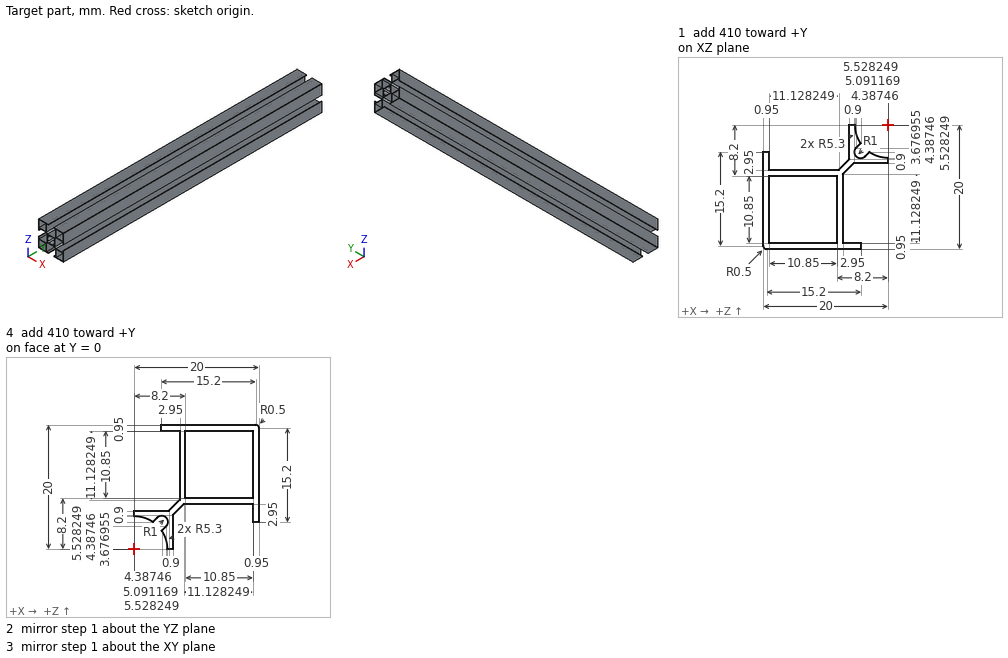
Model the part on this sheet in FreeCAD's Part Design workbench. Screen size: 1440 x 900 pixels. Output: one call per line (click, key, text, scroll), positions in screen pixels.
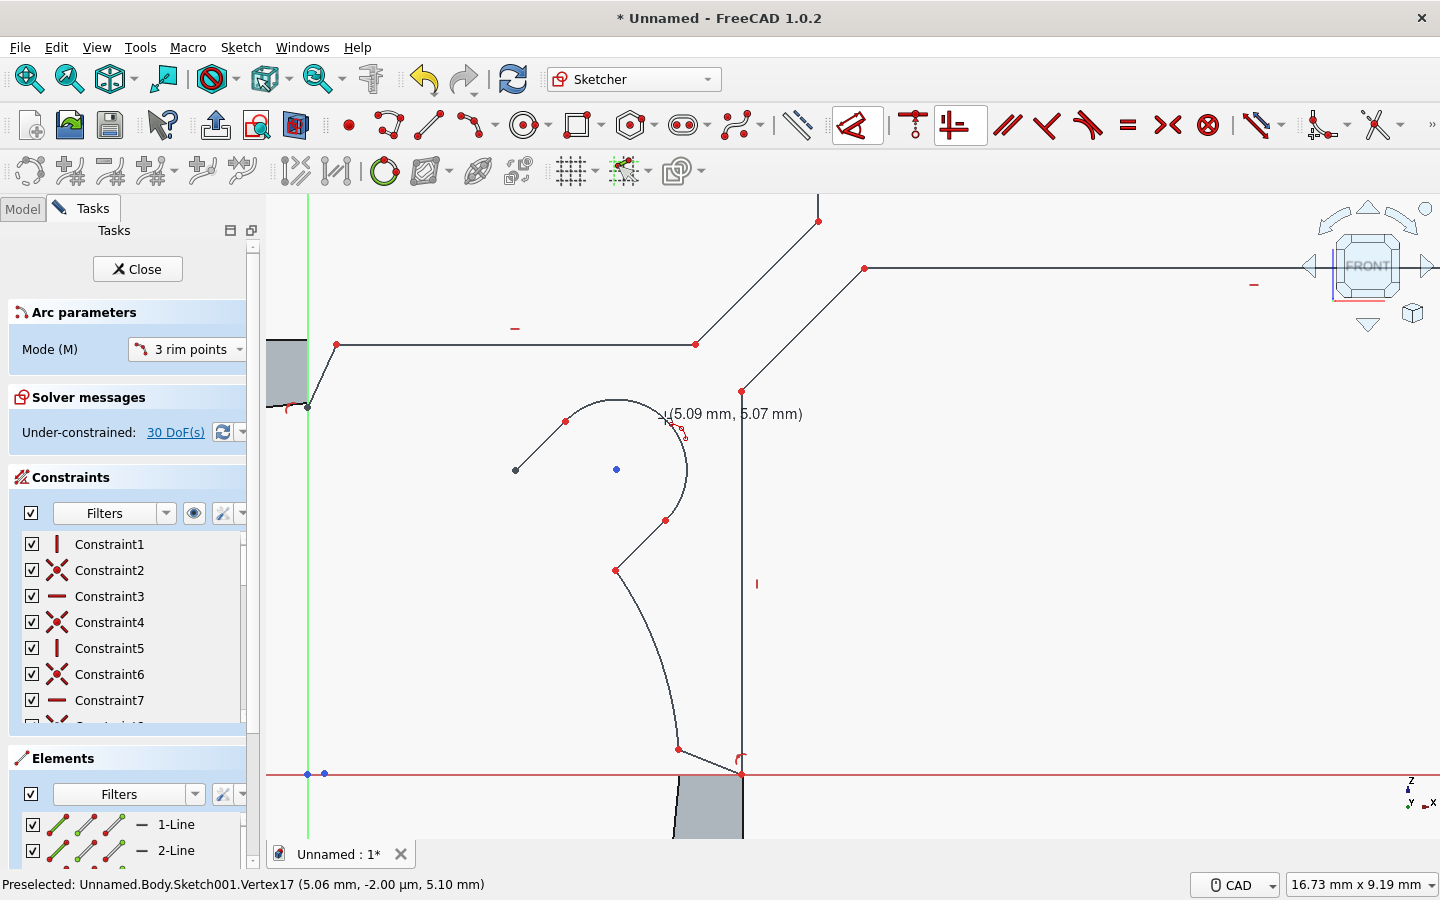
click(516, 471)
click(308, 408)
click(417, 419)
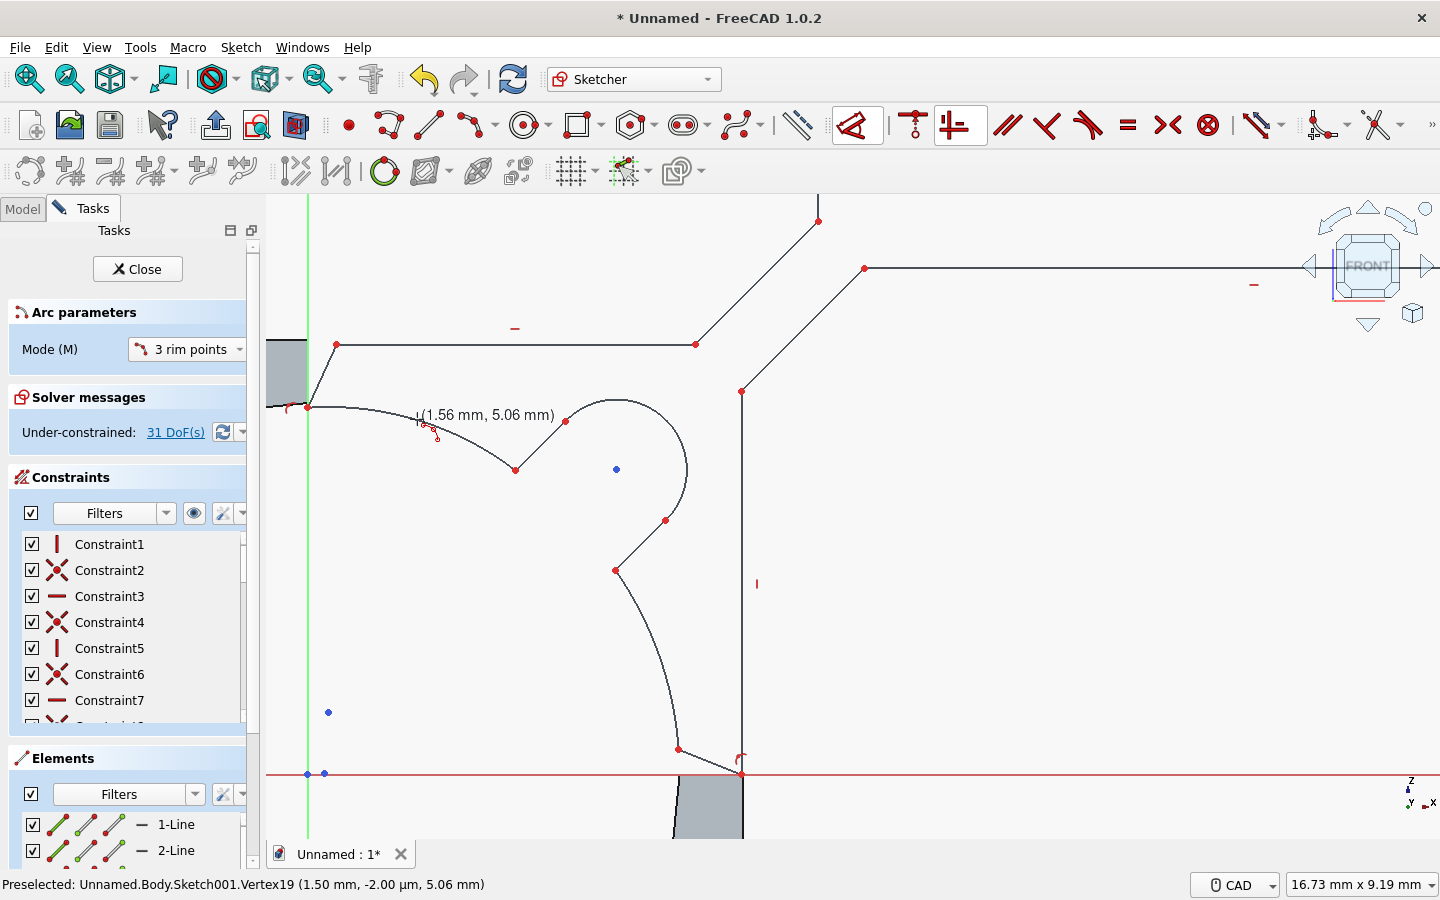
scroll(688, 708, down, 6)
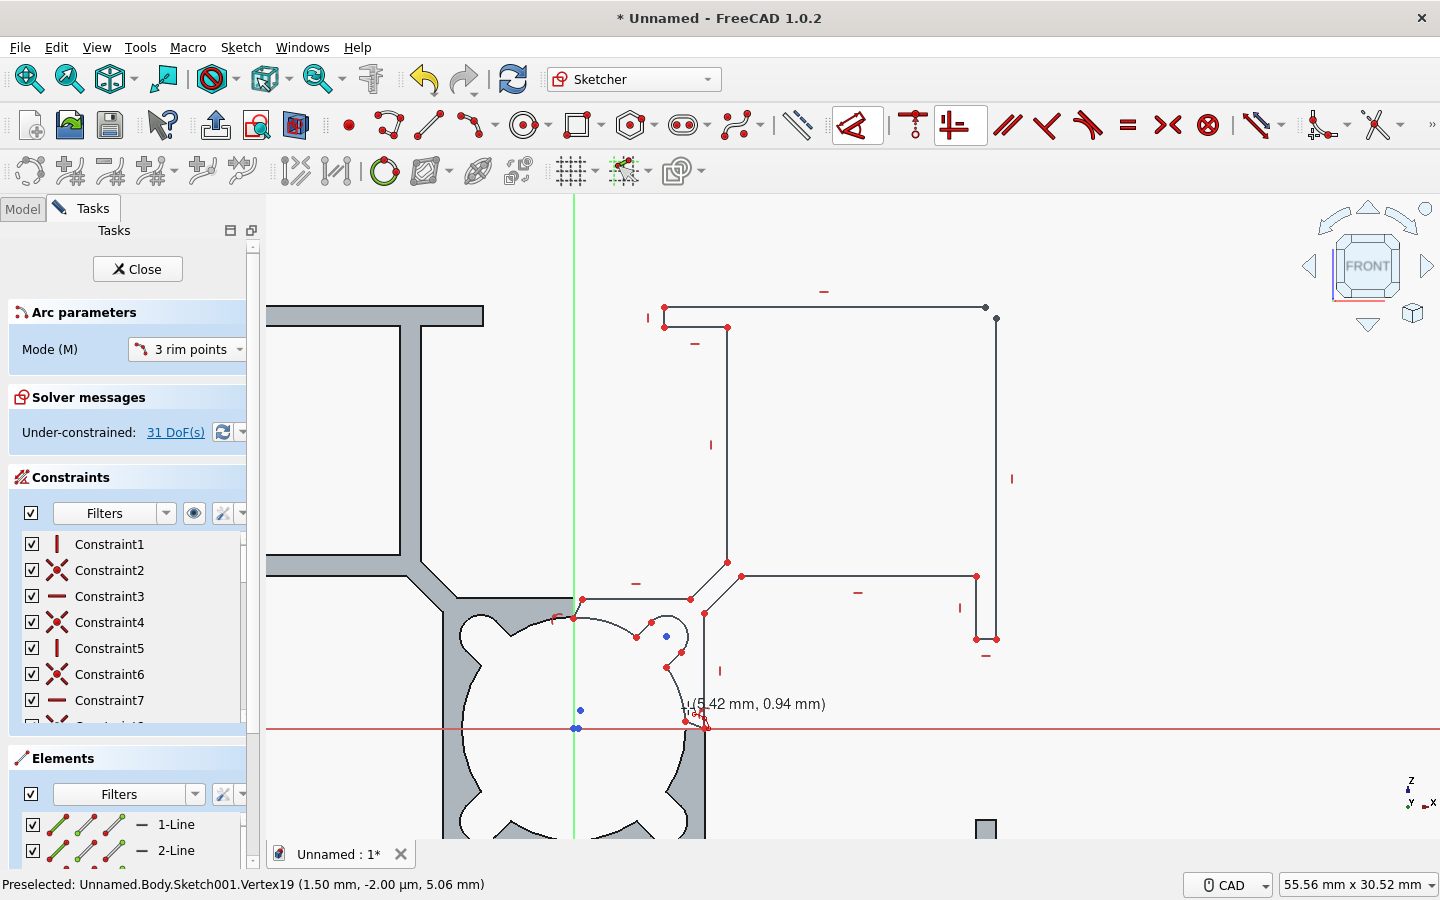
click(985, 307)
click(996, 318)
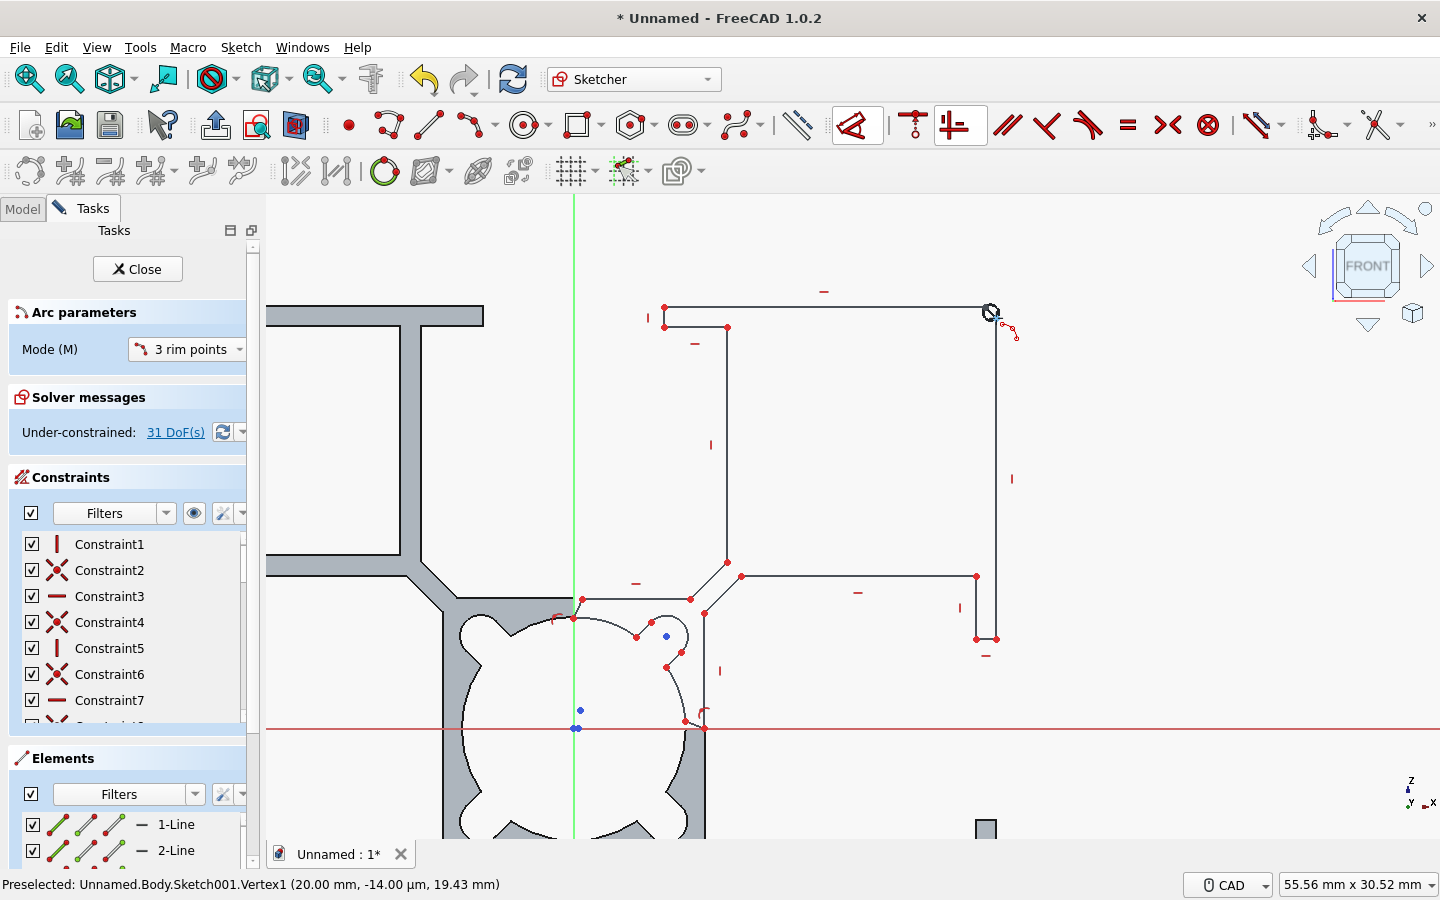
scroll(993, 309, up, 9)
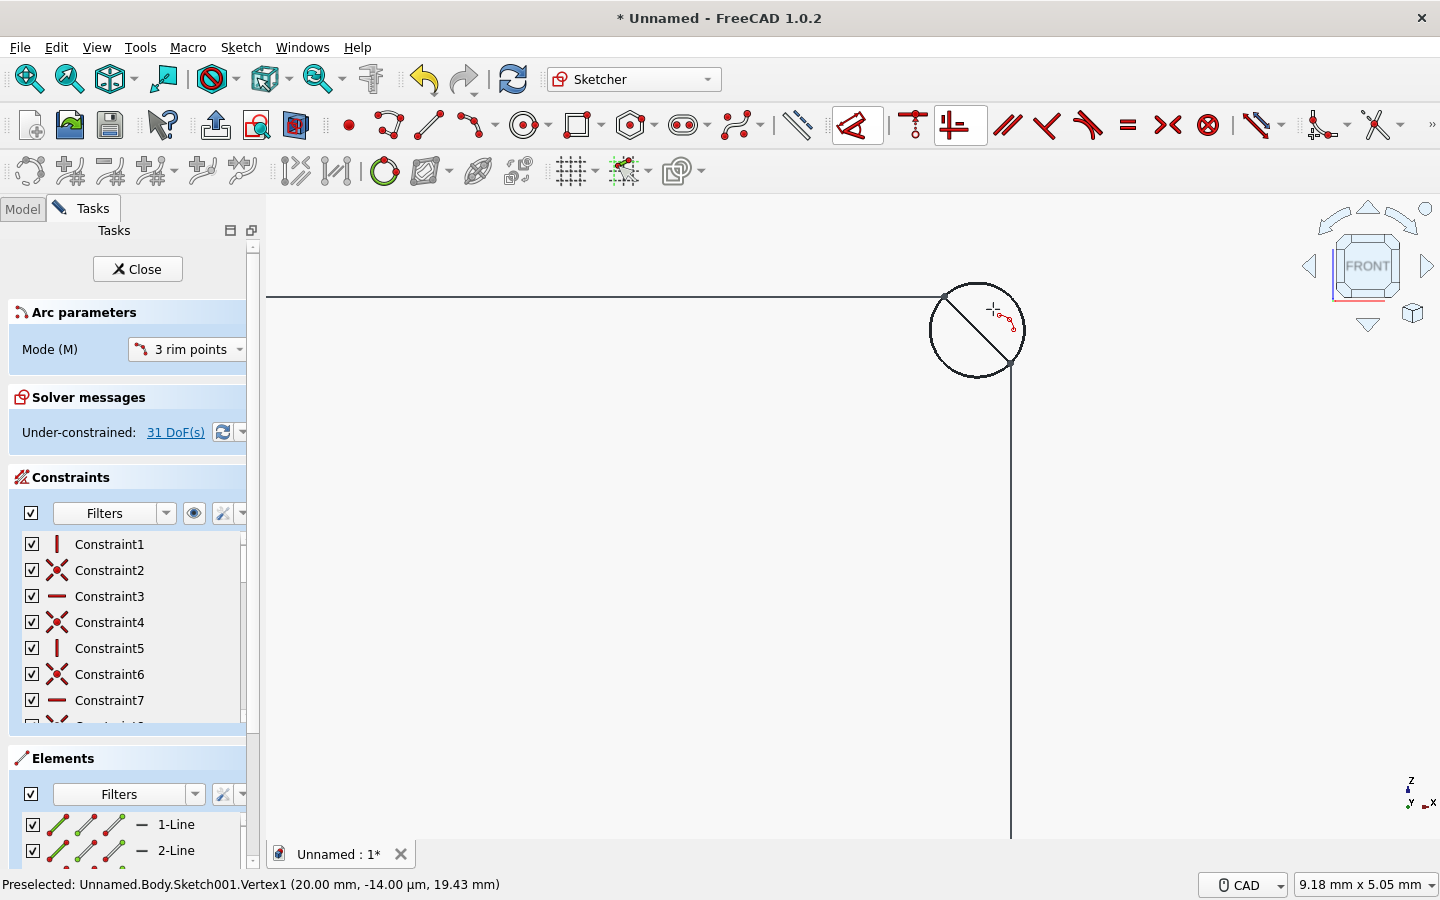
click(991, 309)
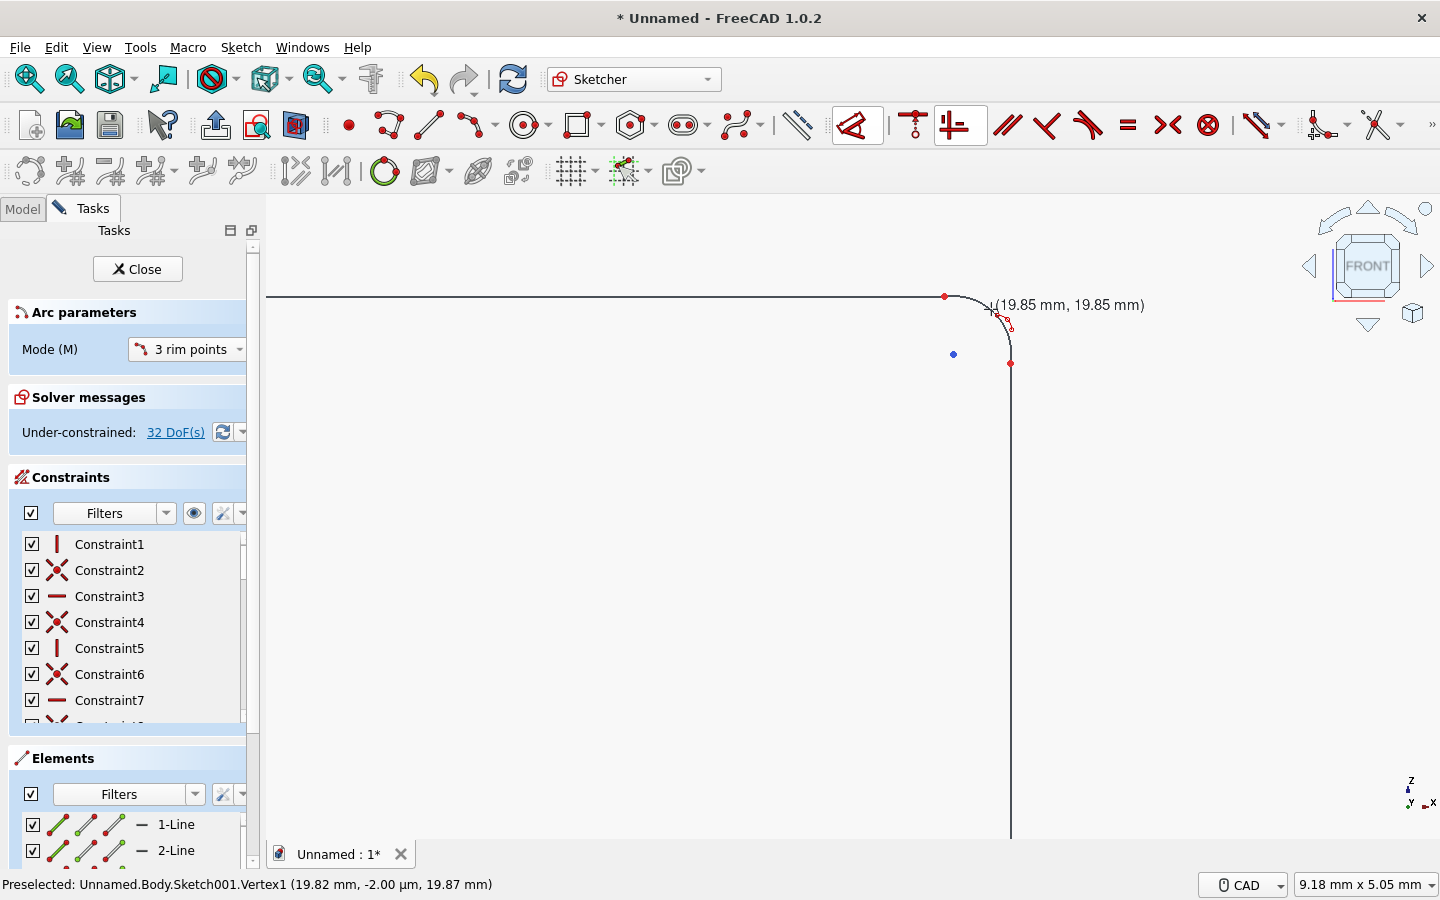
click(578, 126)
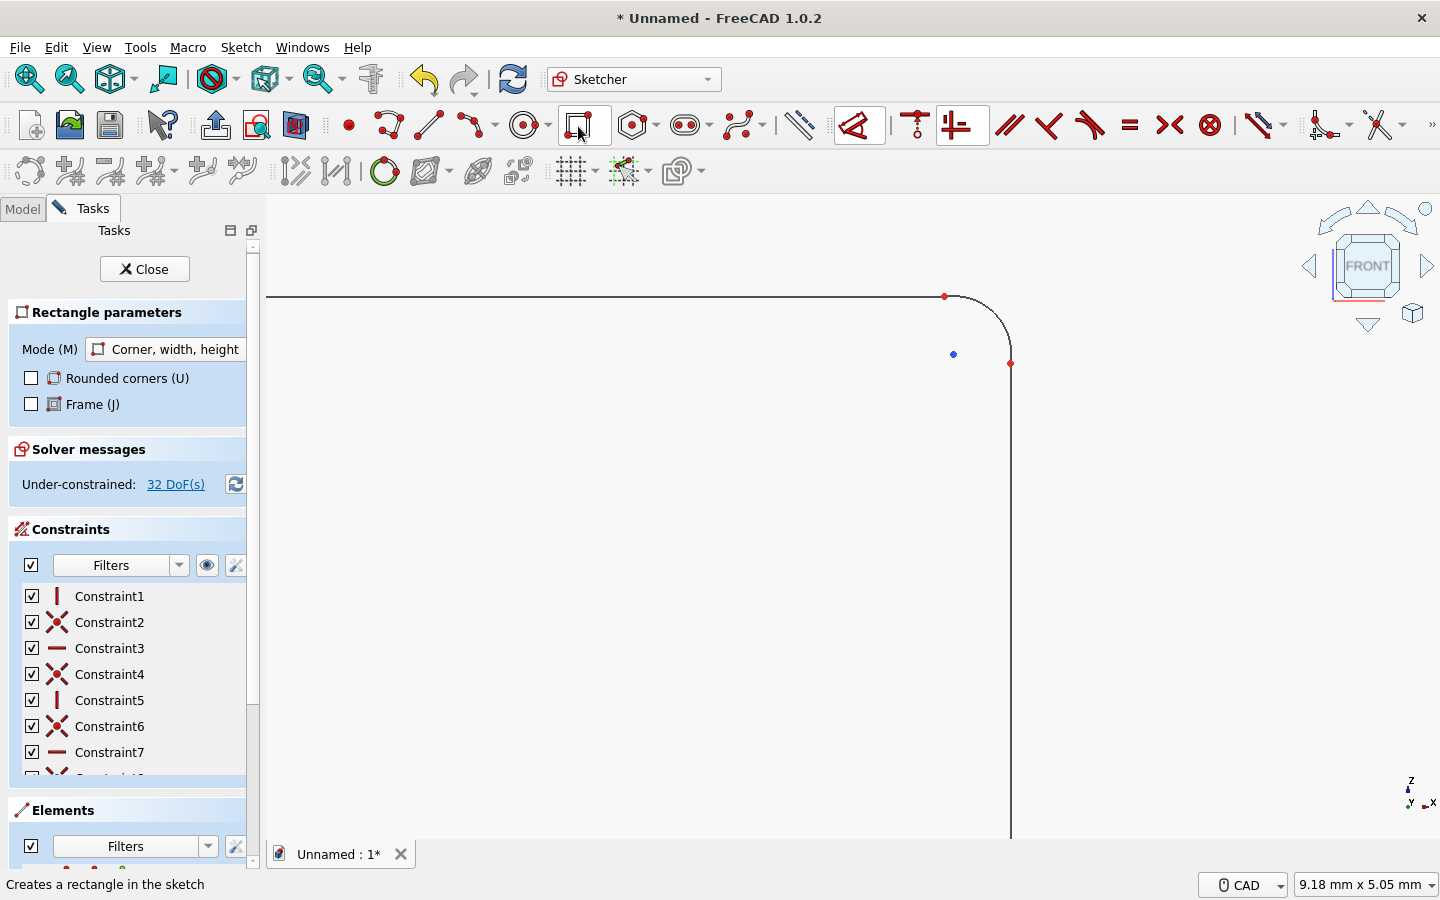
scroll(993, 308, down, 9)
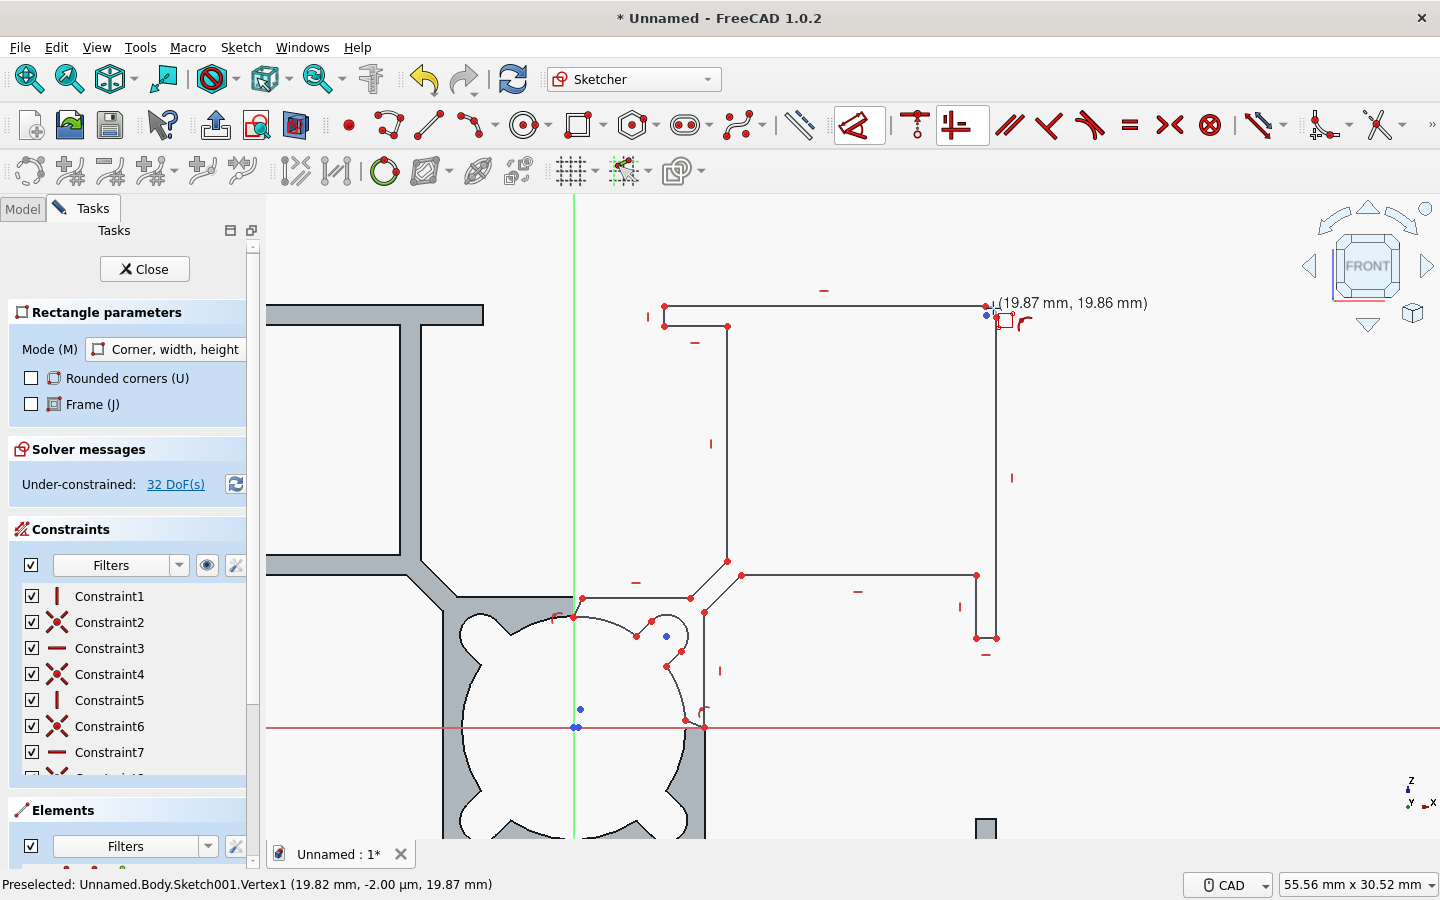
click(747, 325)
click(976, 555)
key(Escape)